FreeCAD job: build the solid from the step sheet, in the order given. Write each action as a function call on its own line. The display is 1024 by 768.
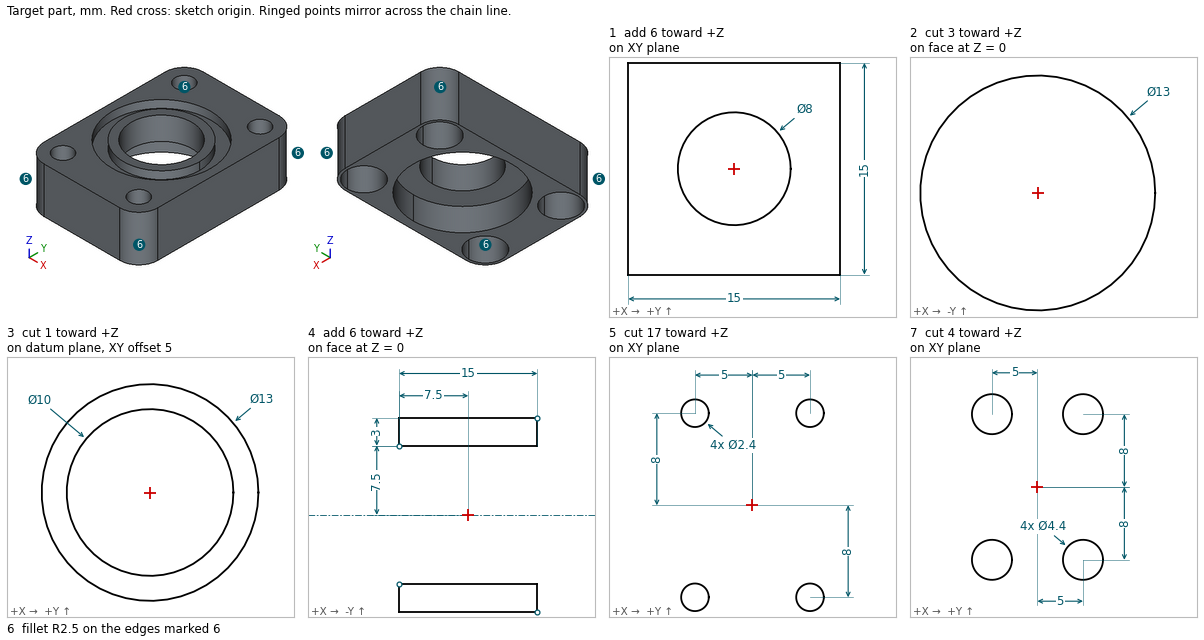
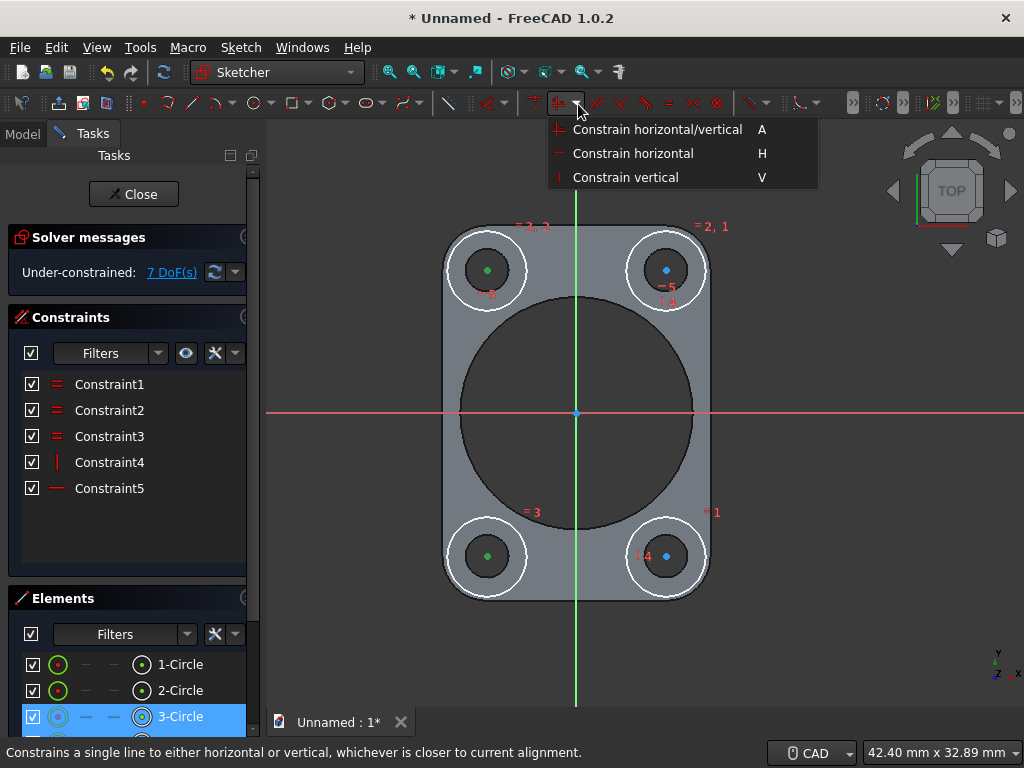
click(683, 177)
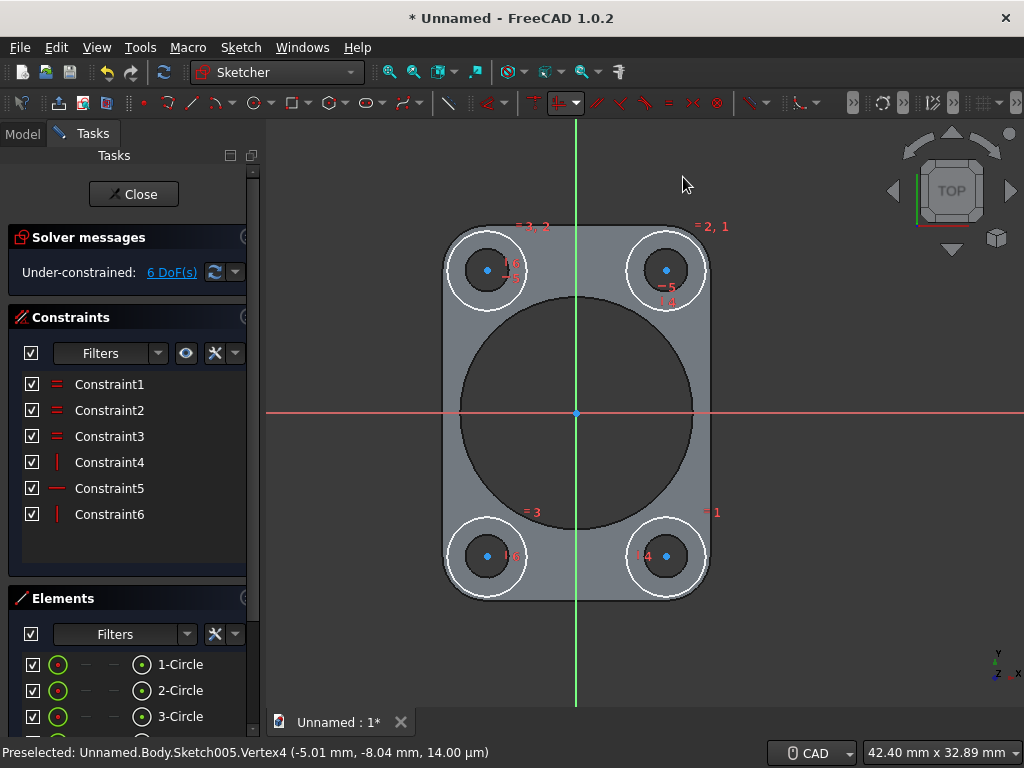
click(666, 557)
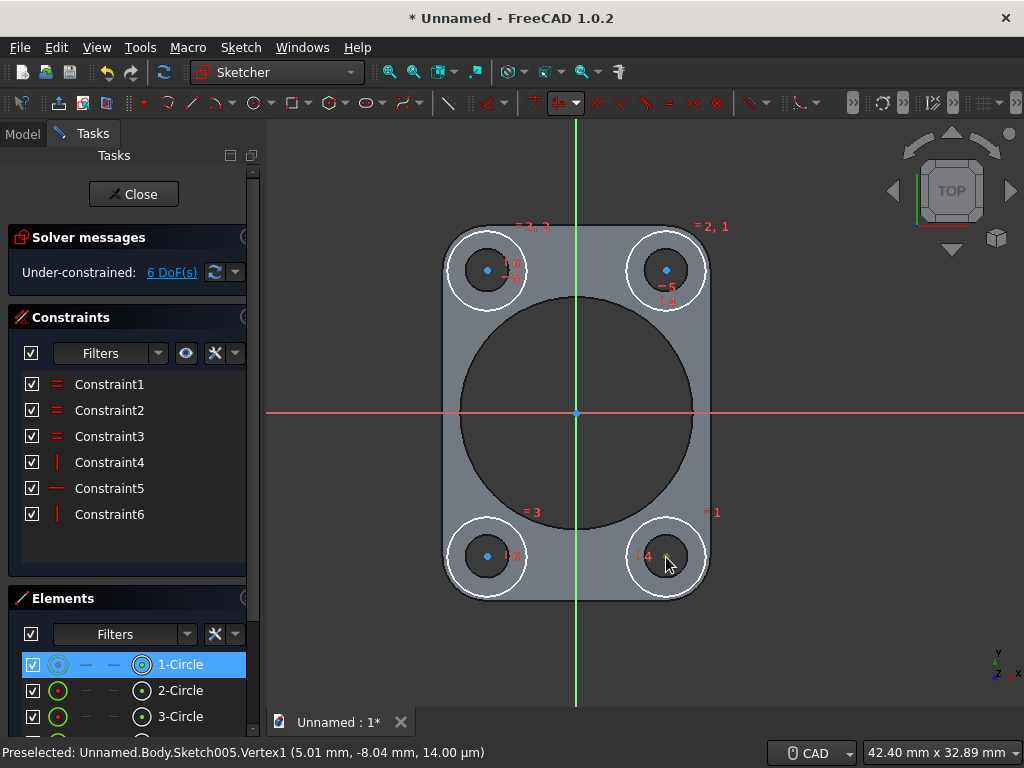
click(487, 557)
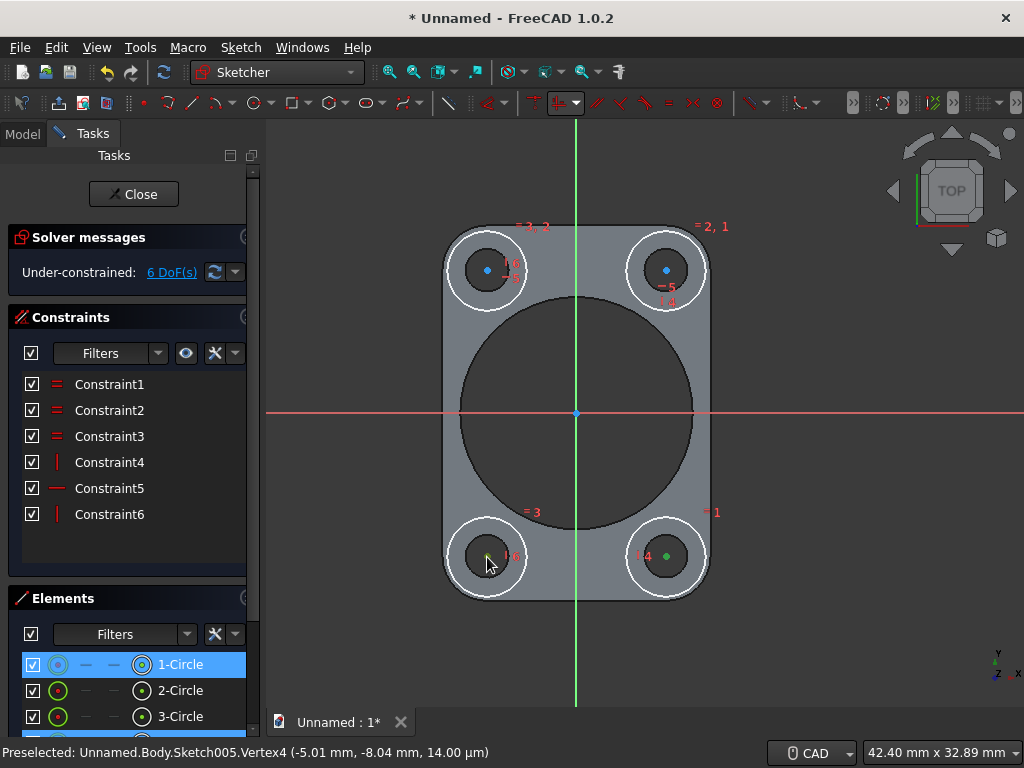
key(h)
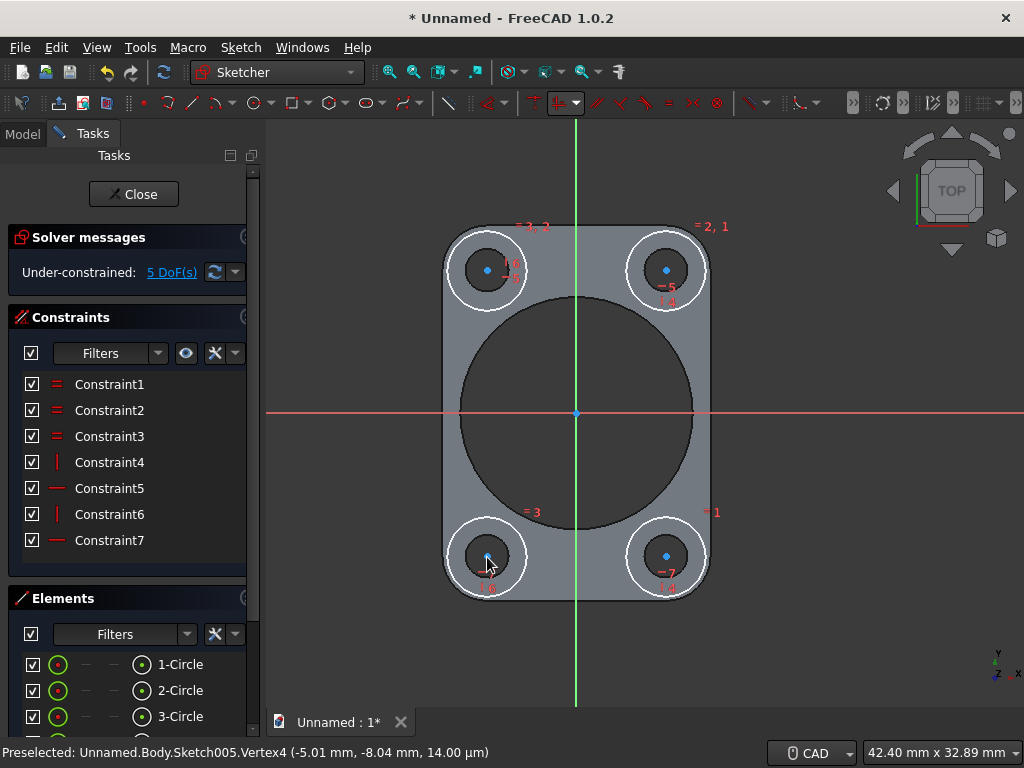
key(d)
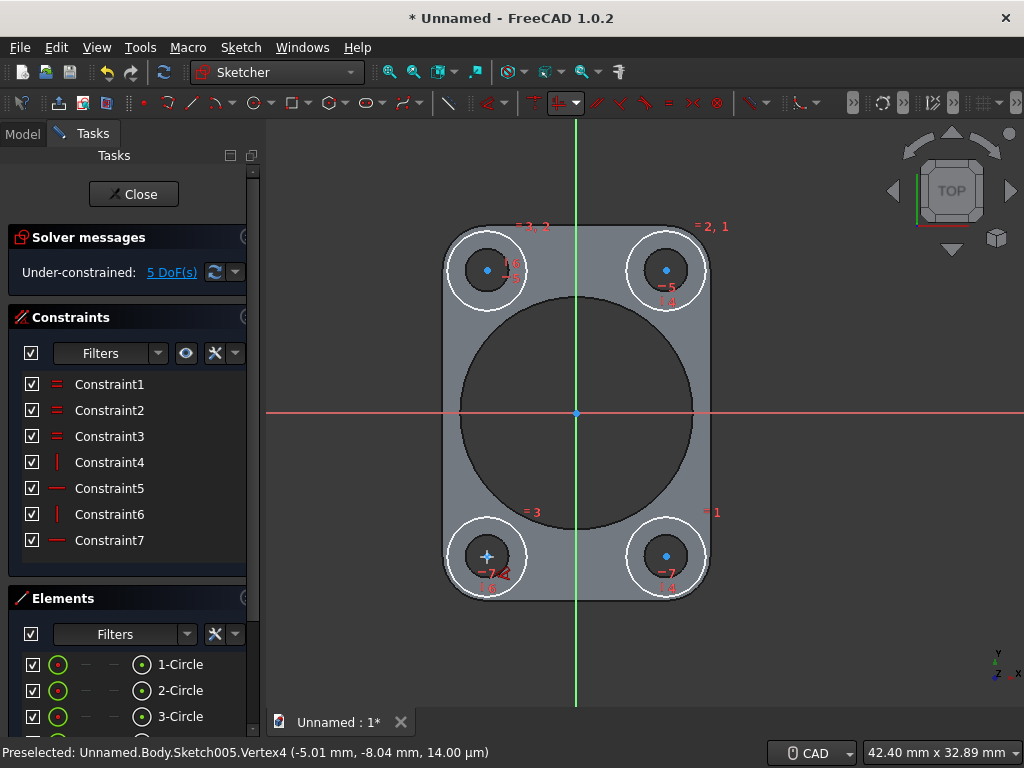
click(694, 529)
click(717, 506)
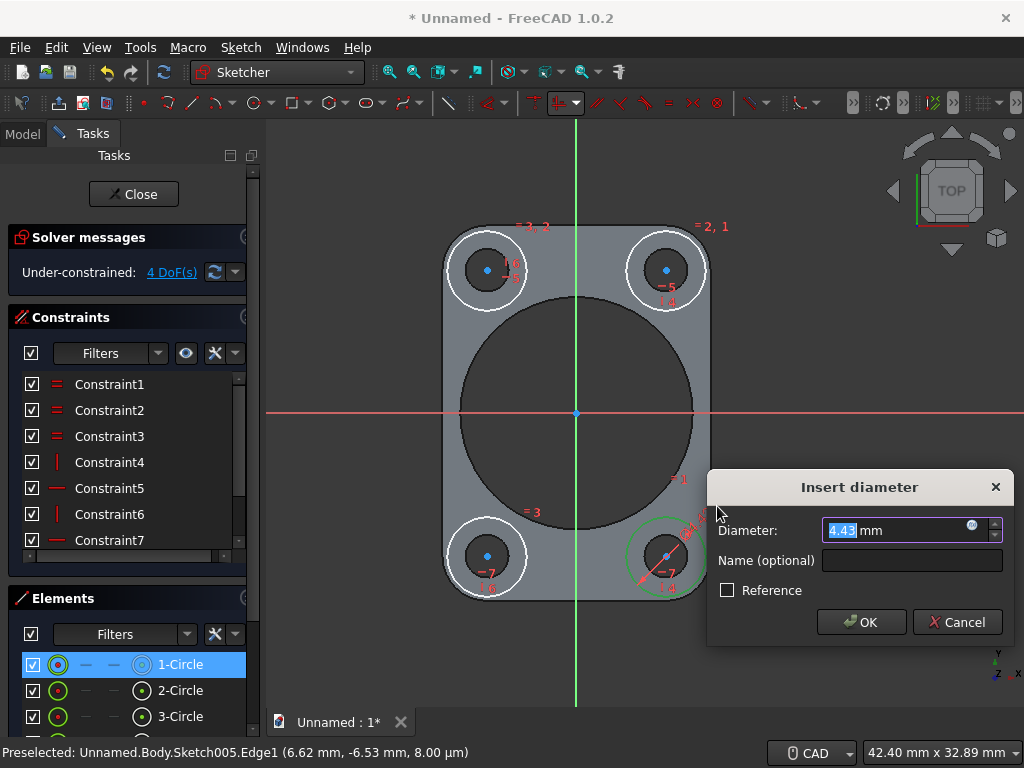
text(4.4)
key(Return)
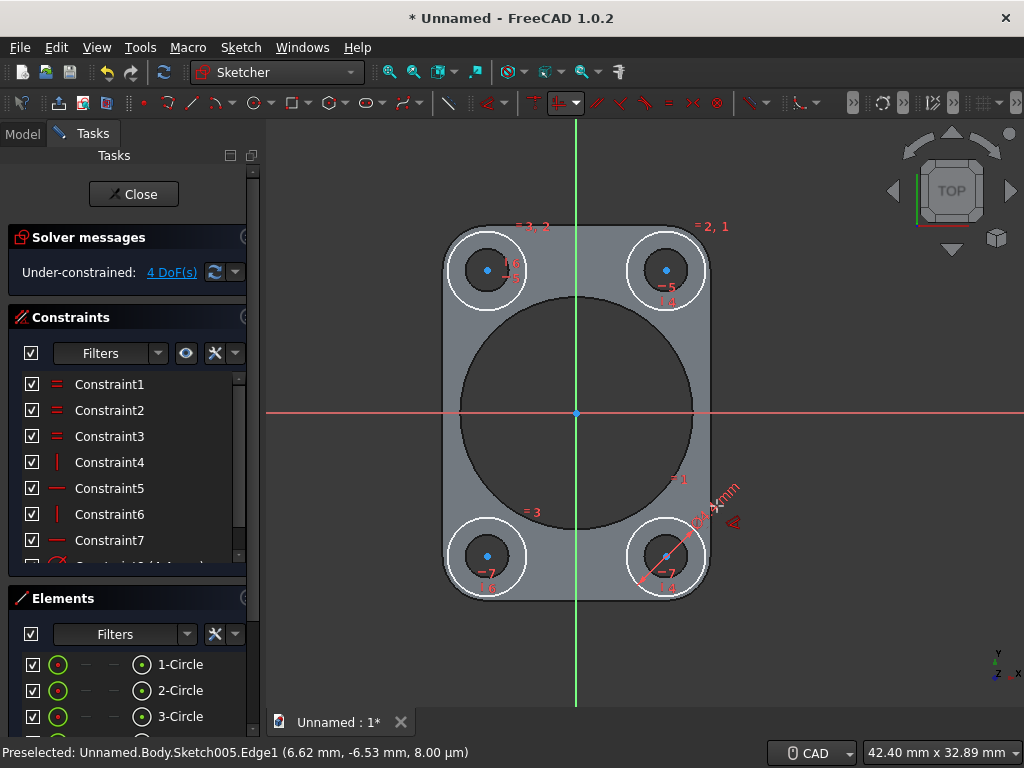
click(666, 557)
click(621, 591)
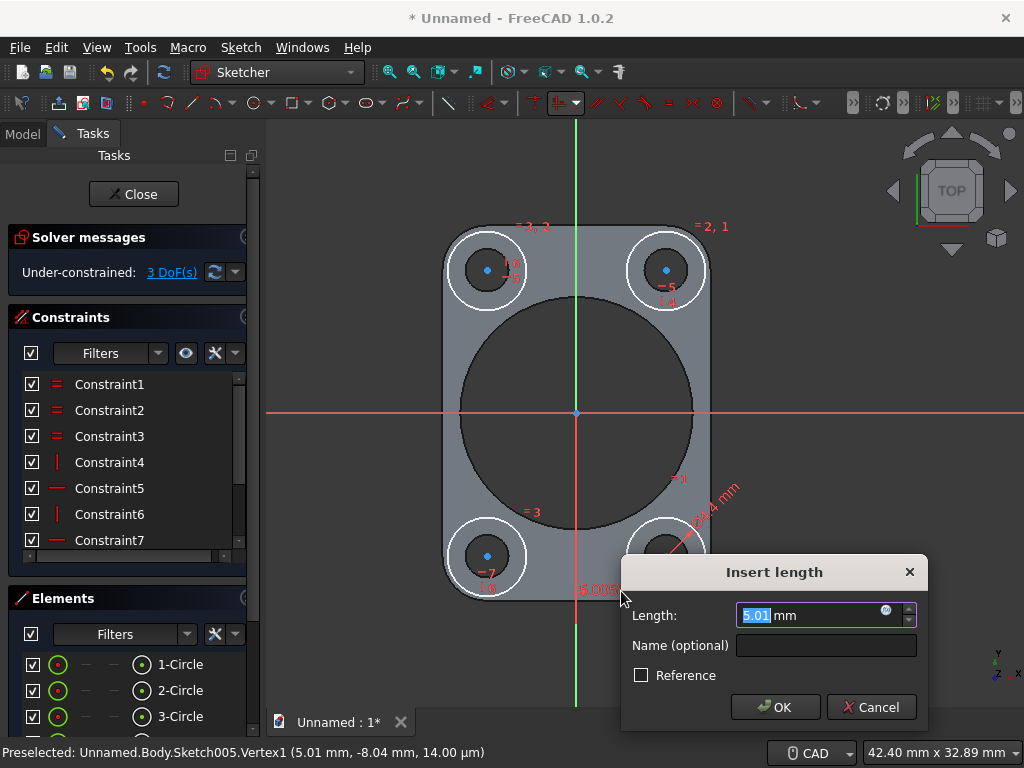
text(5)
key(Return)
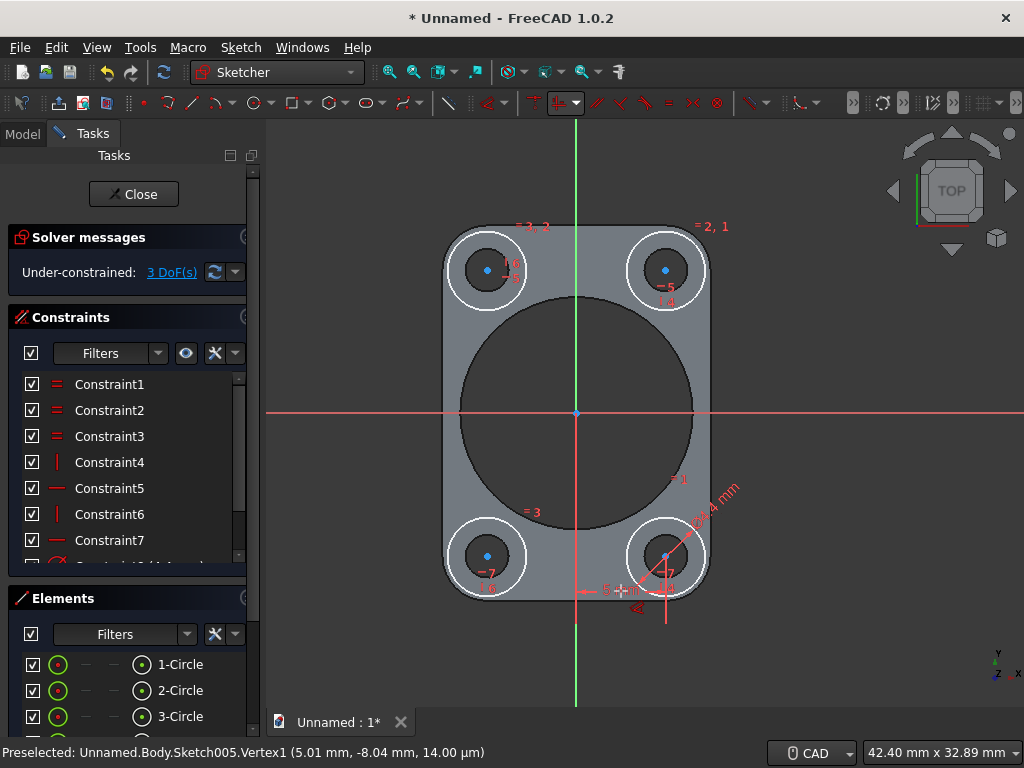
click(666, 557)
click(700, 485)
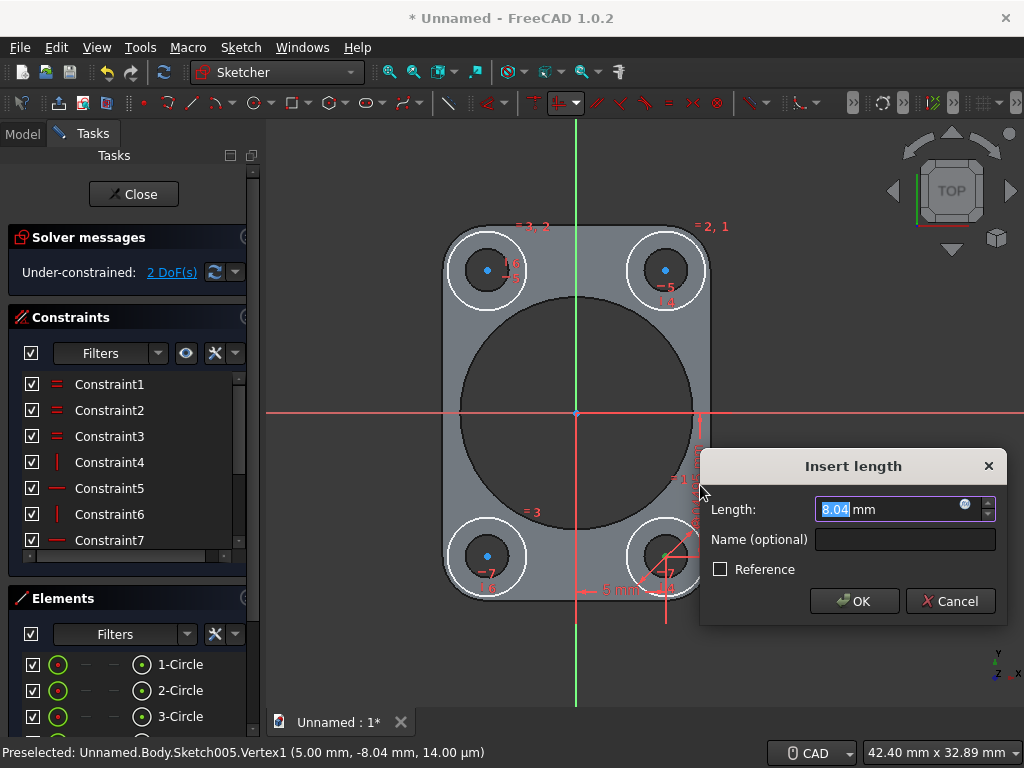
text(8)
key(Return)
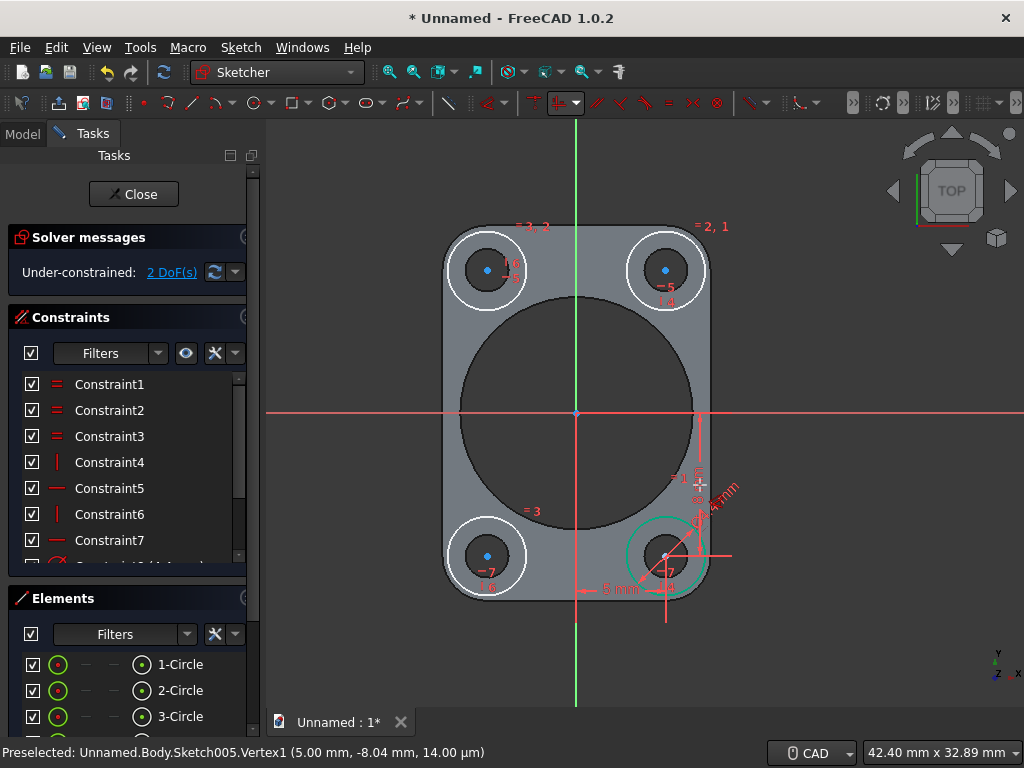
click(666, 271)
click(700, 342)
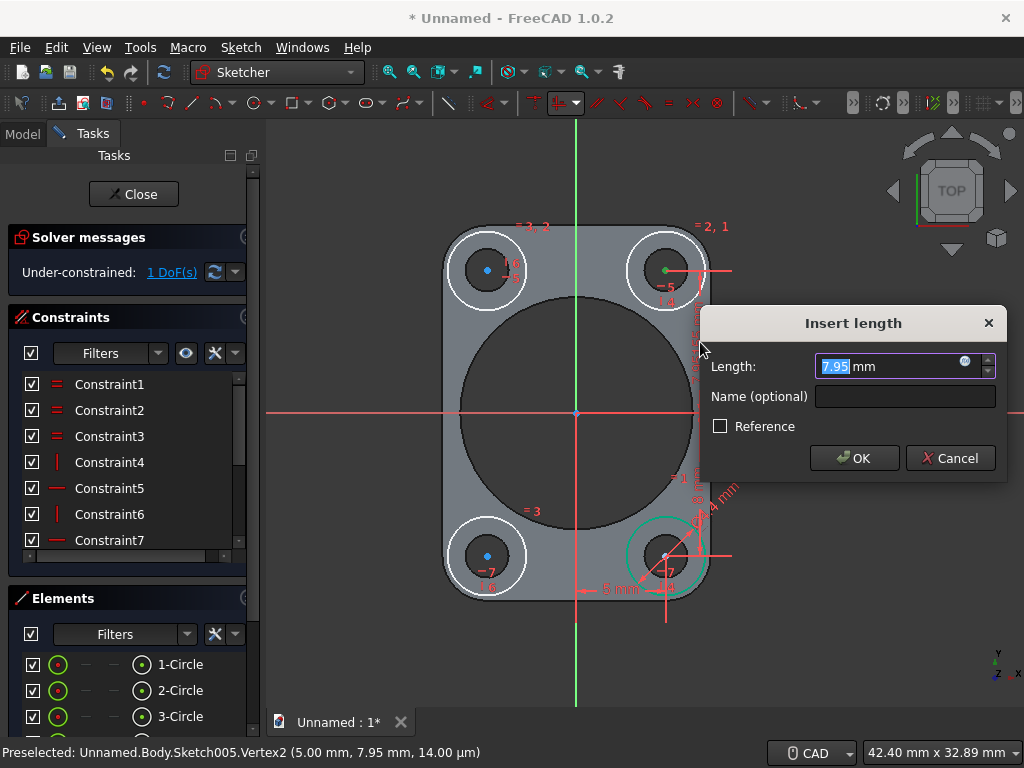
text(8)
key(Return)